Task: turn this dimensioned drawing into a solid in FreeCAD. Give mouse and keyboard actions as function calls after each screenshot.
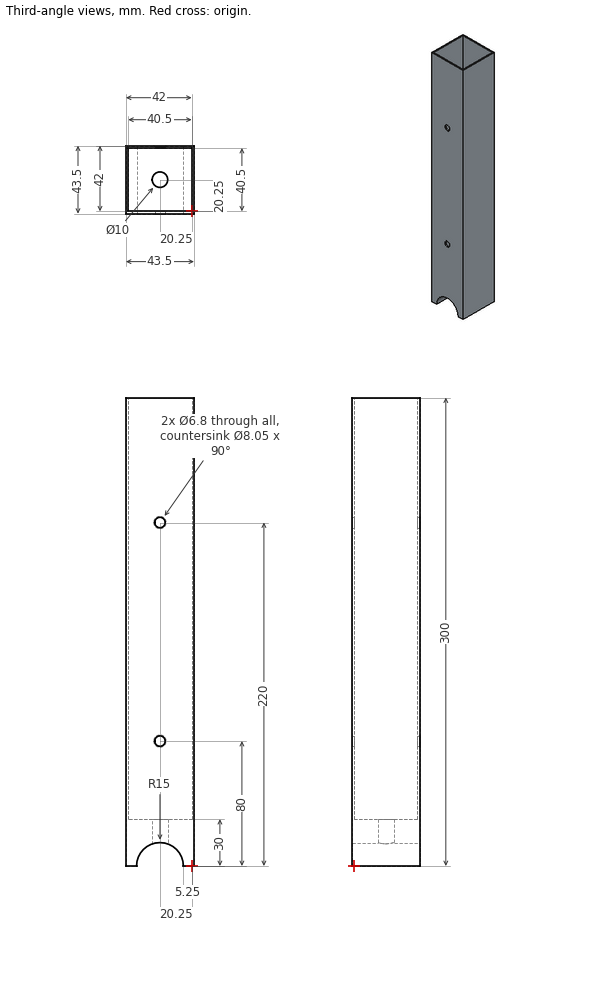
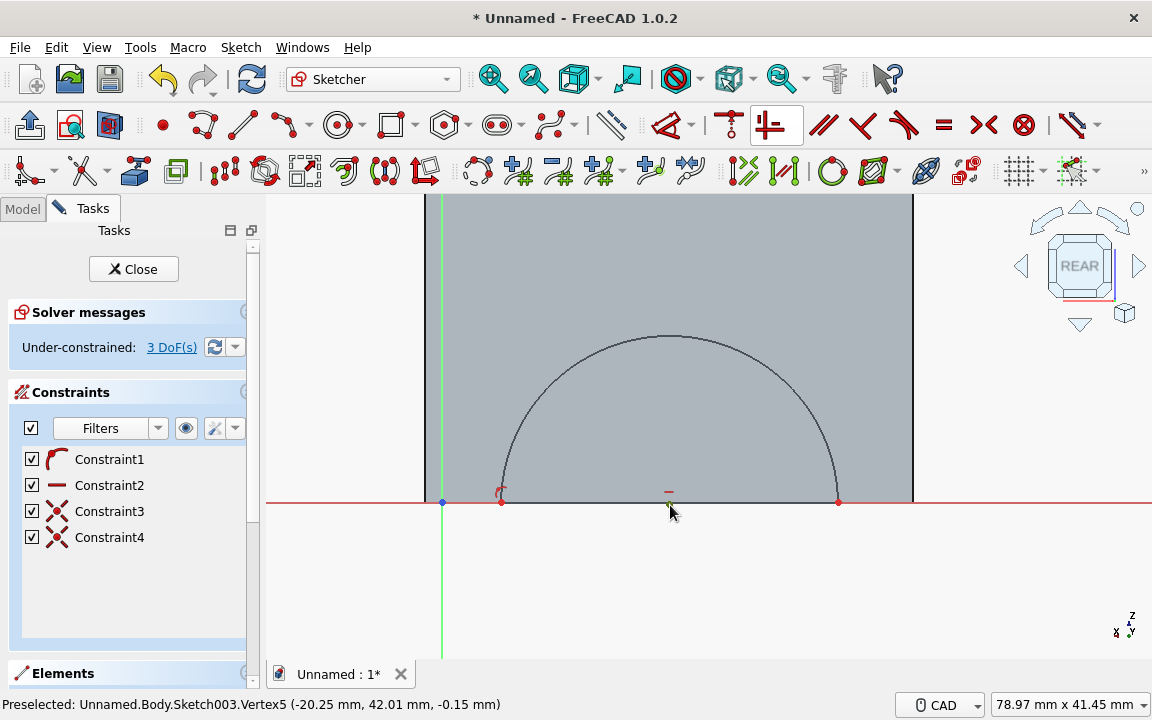
click(344, 503)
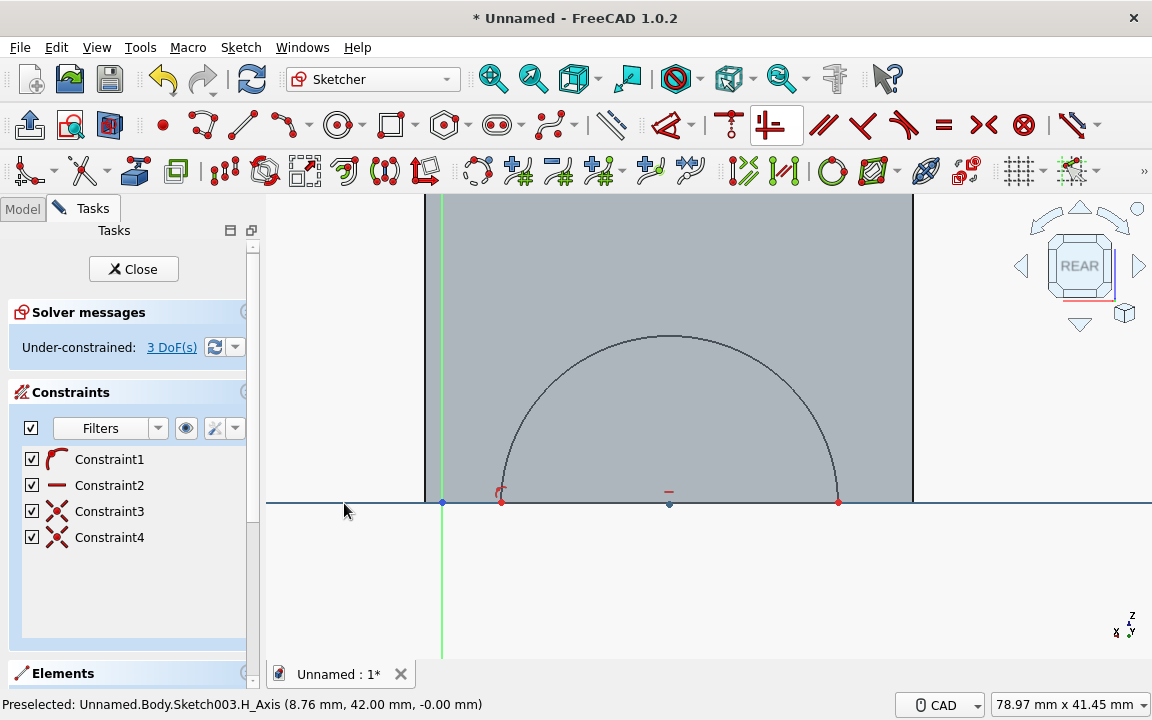
click(730, 126)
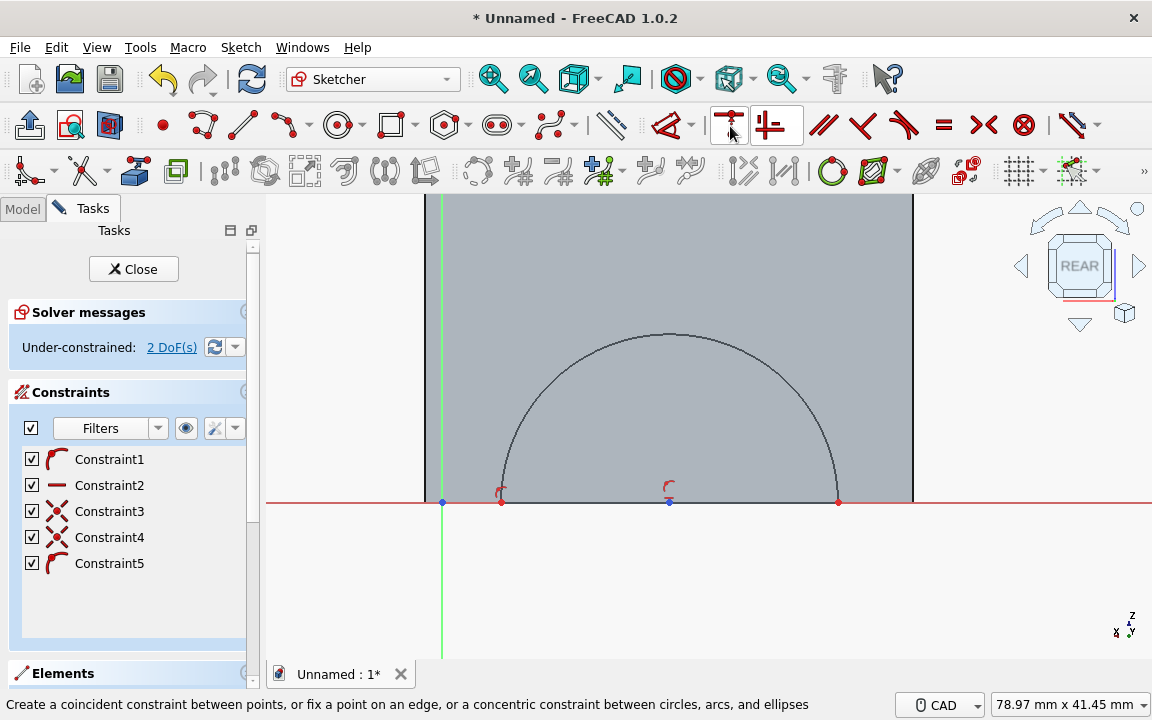
click(666, 126)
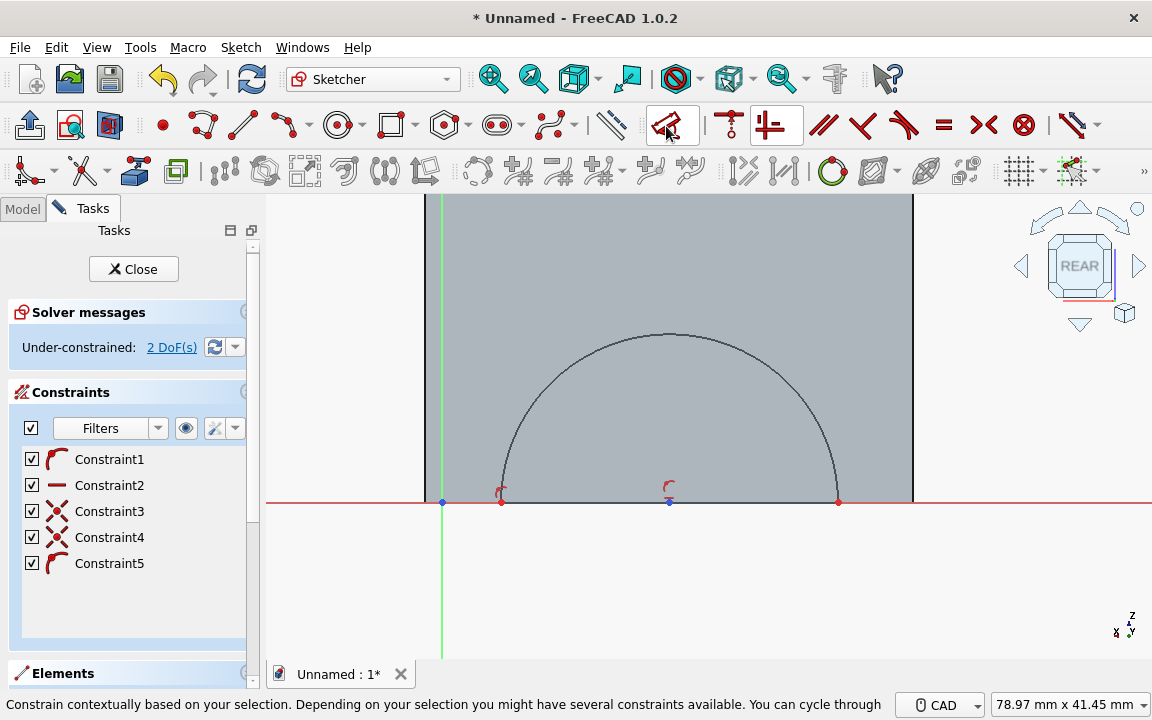
click(769, 366)
click(788, 340)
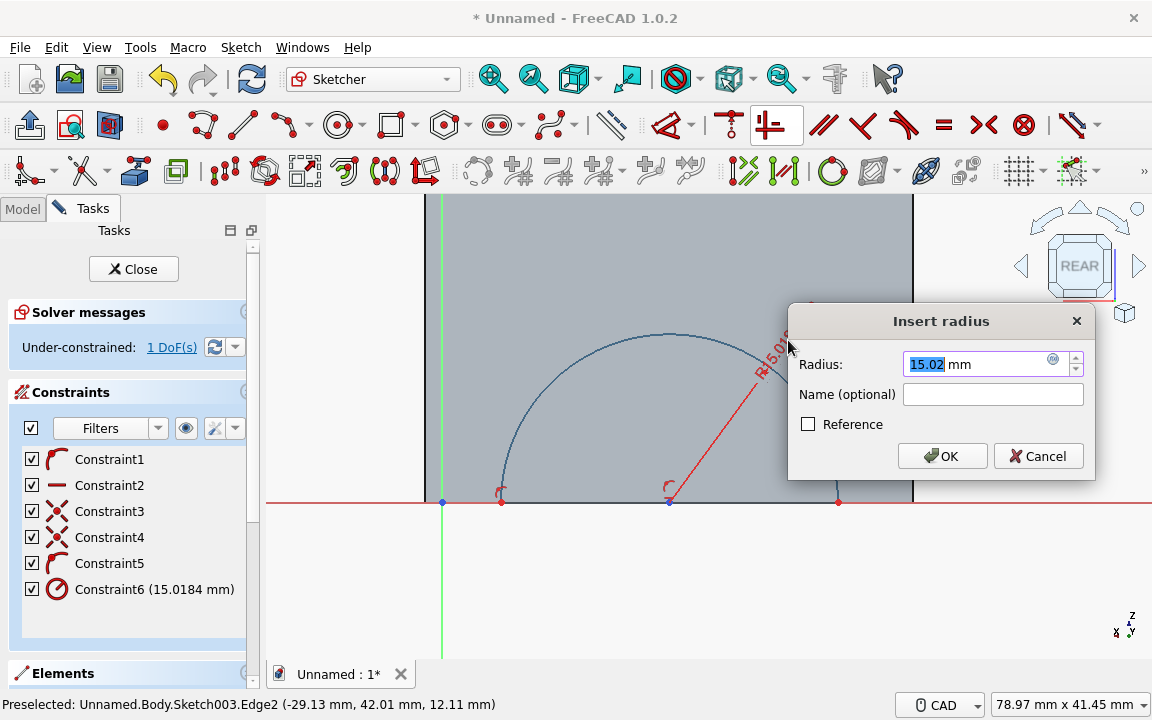
text(15)
key(Return)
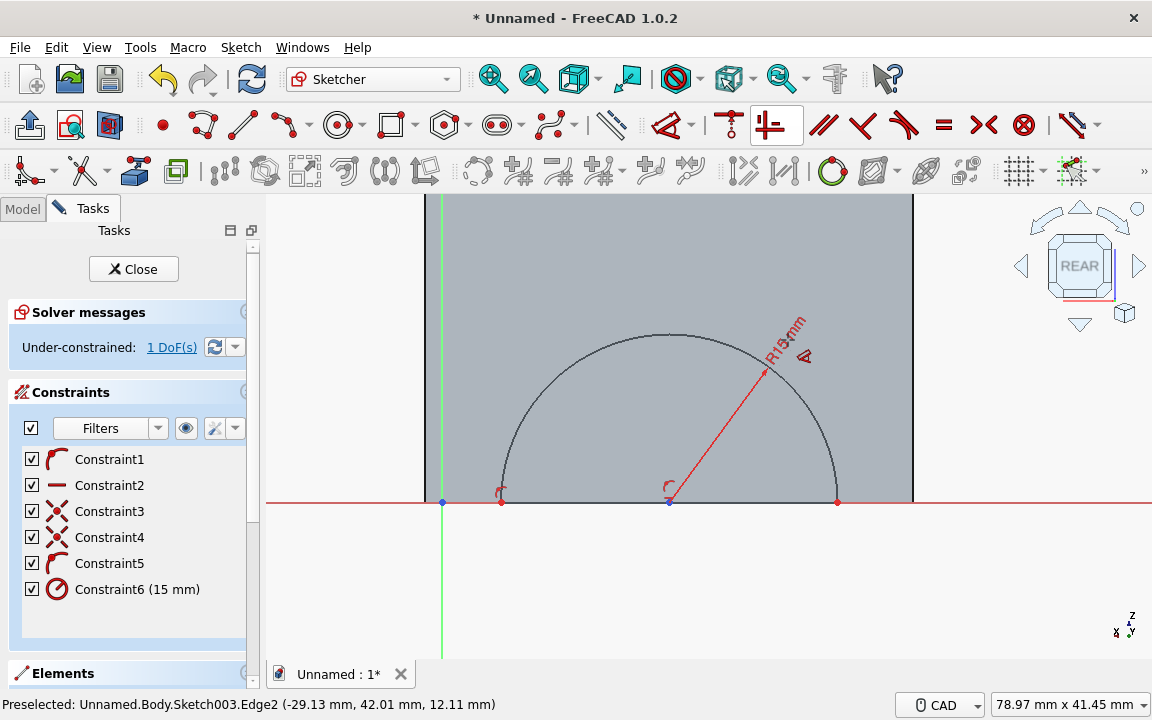
click(501, 503)
click(472, 537)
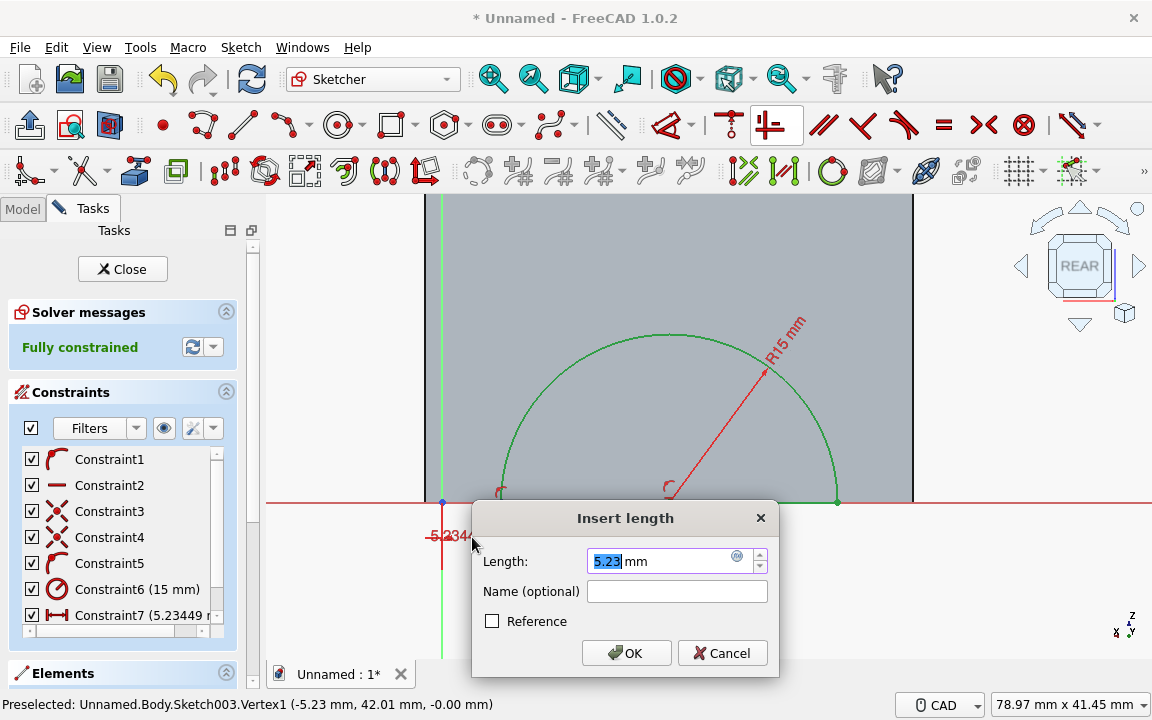
text(5.25)
key(Return)
key(Escape)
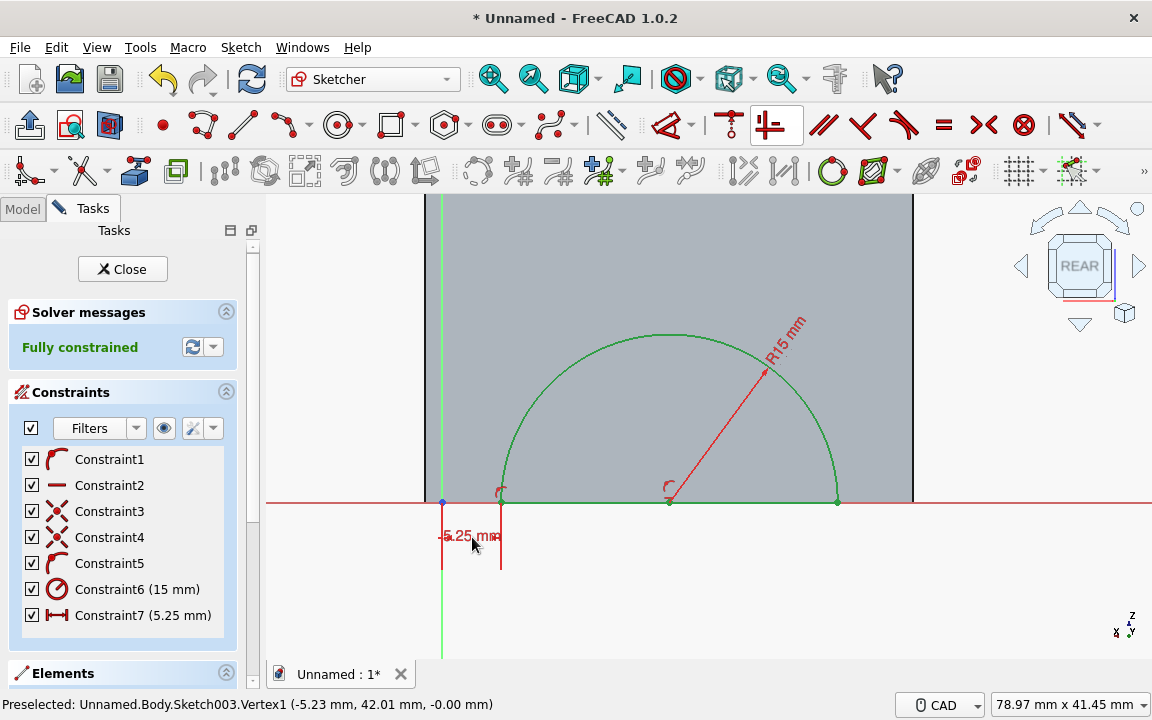
click(123, 269)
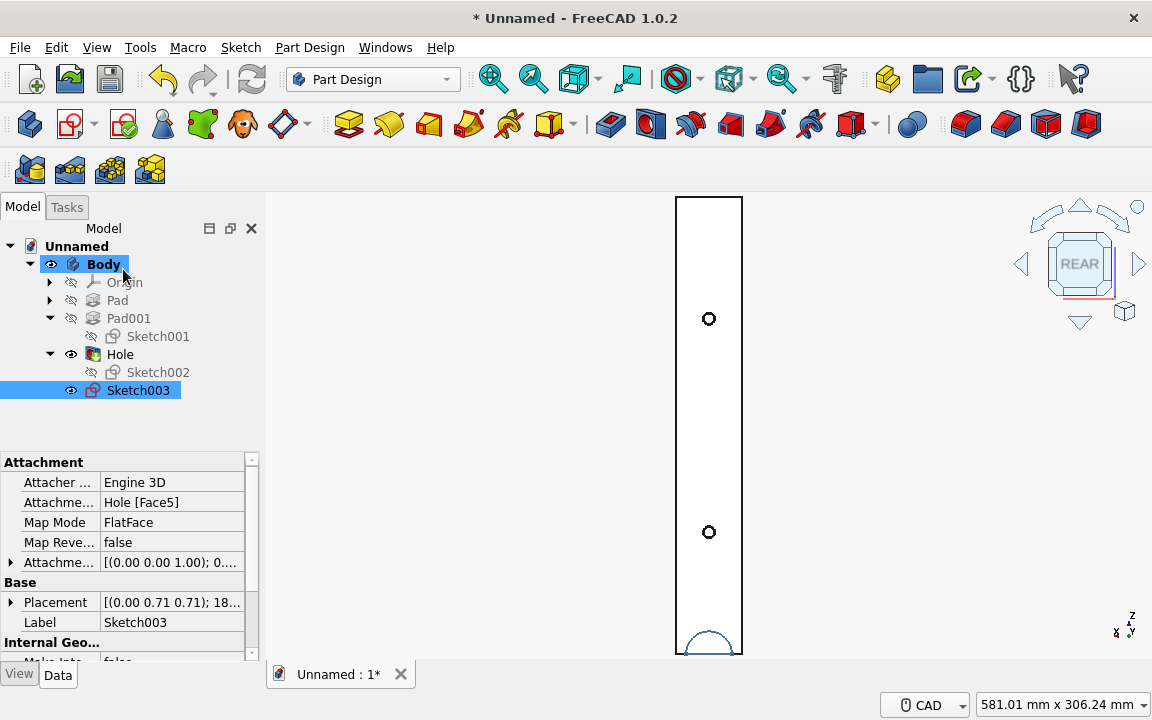
click(612, 124)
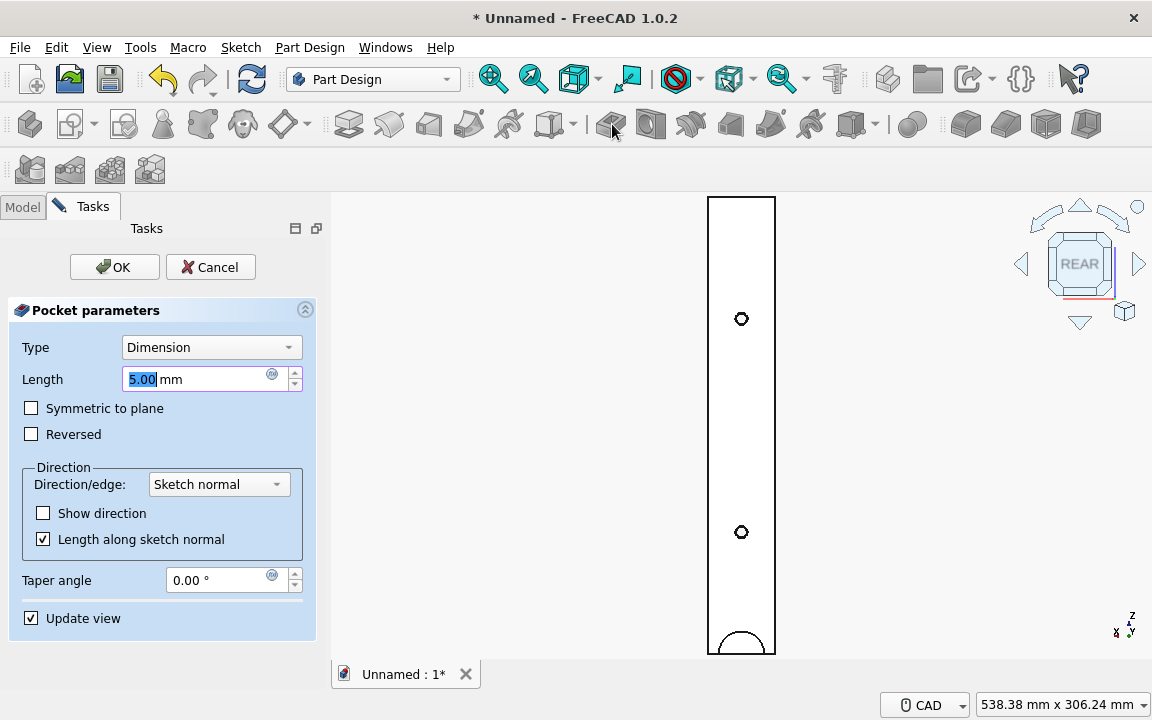
click(212, 348)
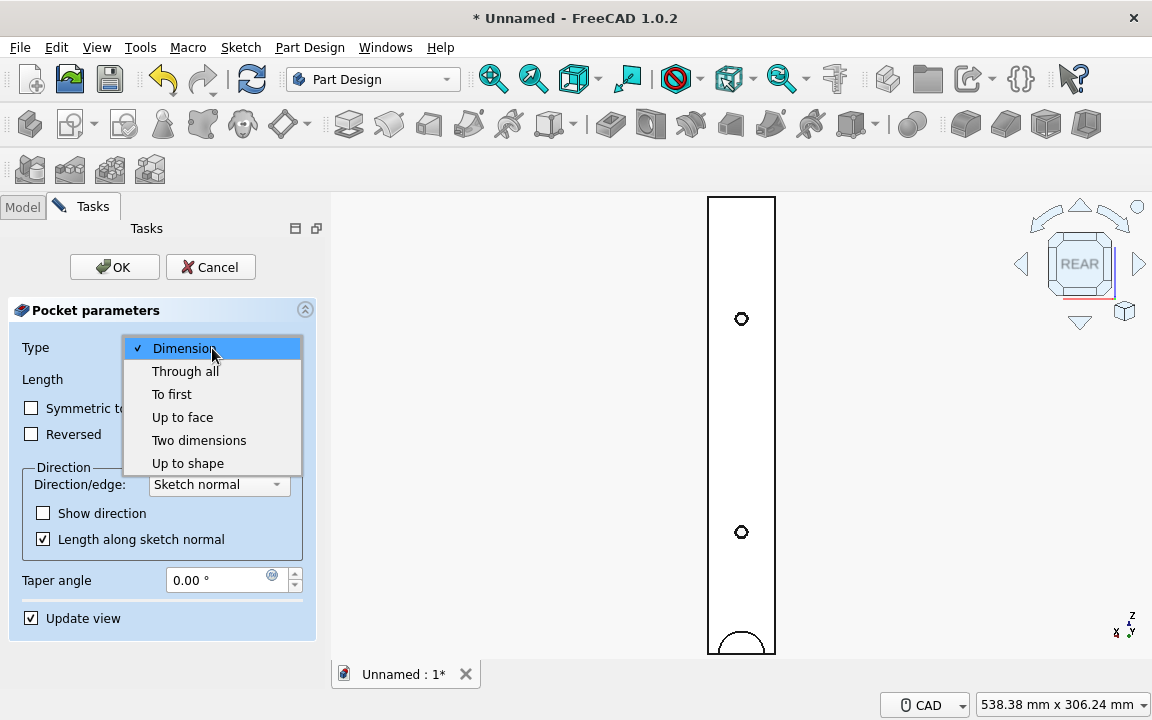
click(212, 372)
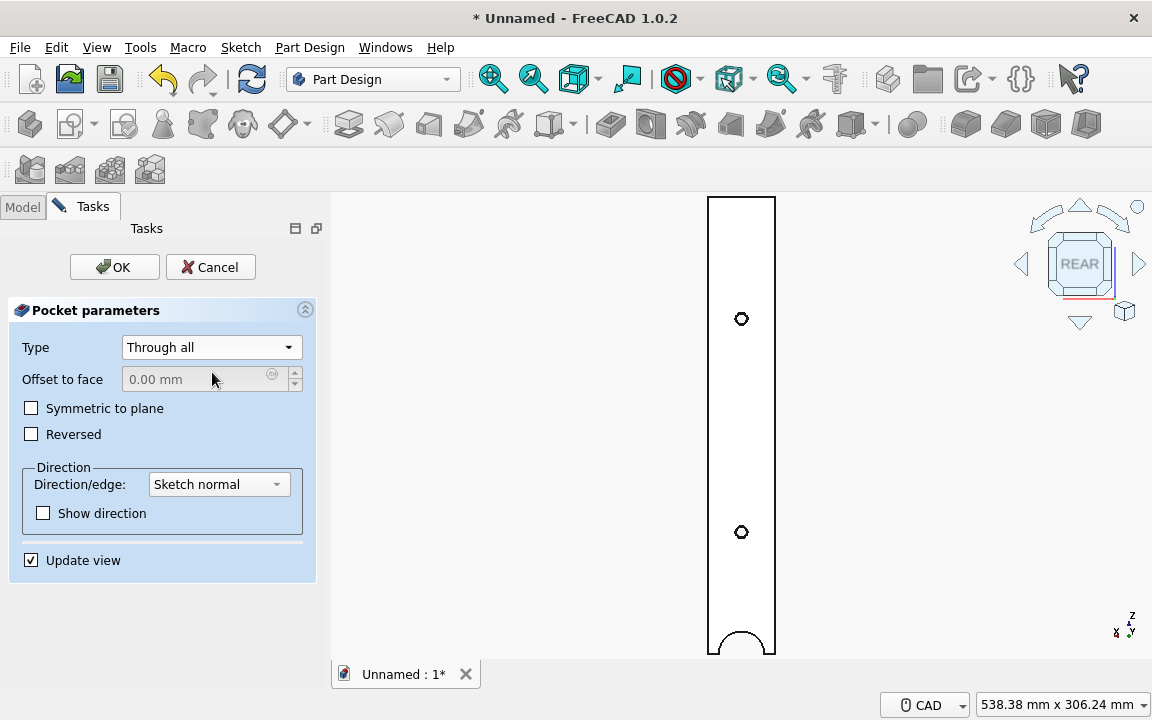
click(115, 267)